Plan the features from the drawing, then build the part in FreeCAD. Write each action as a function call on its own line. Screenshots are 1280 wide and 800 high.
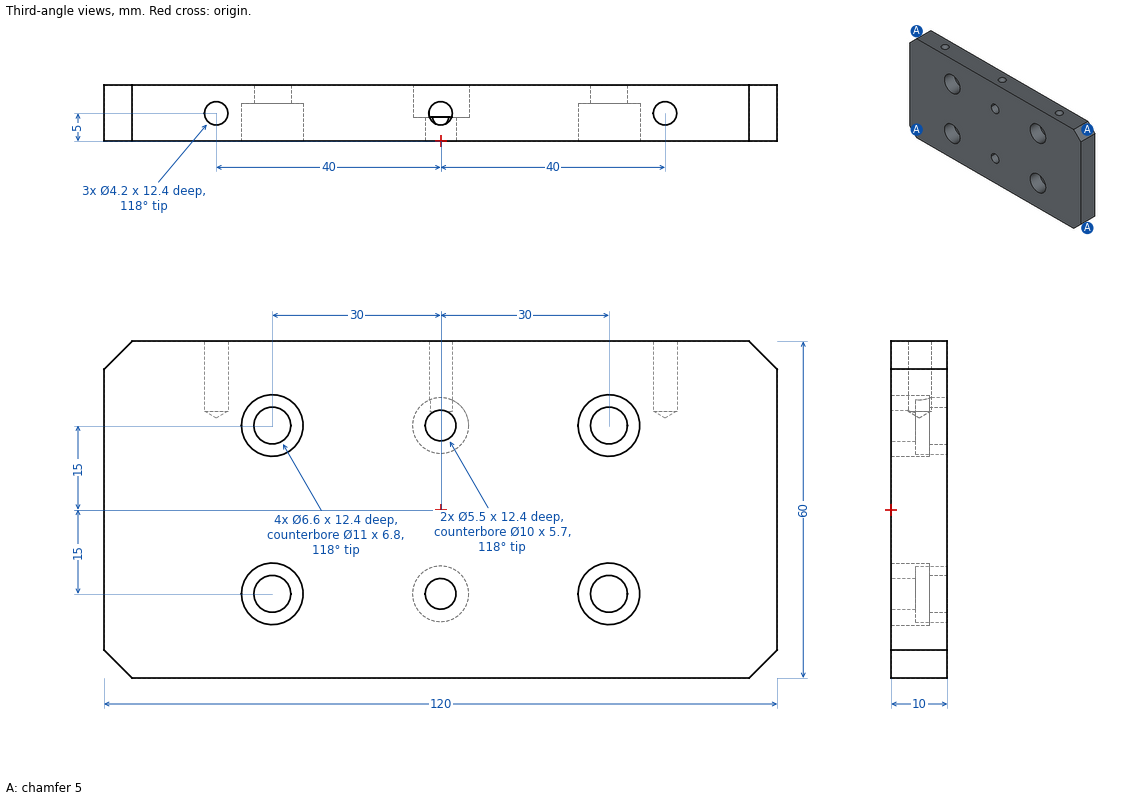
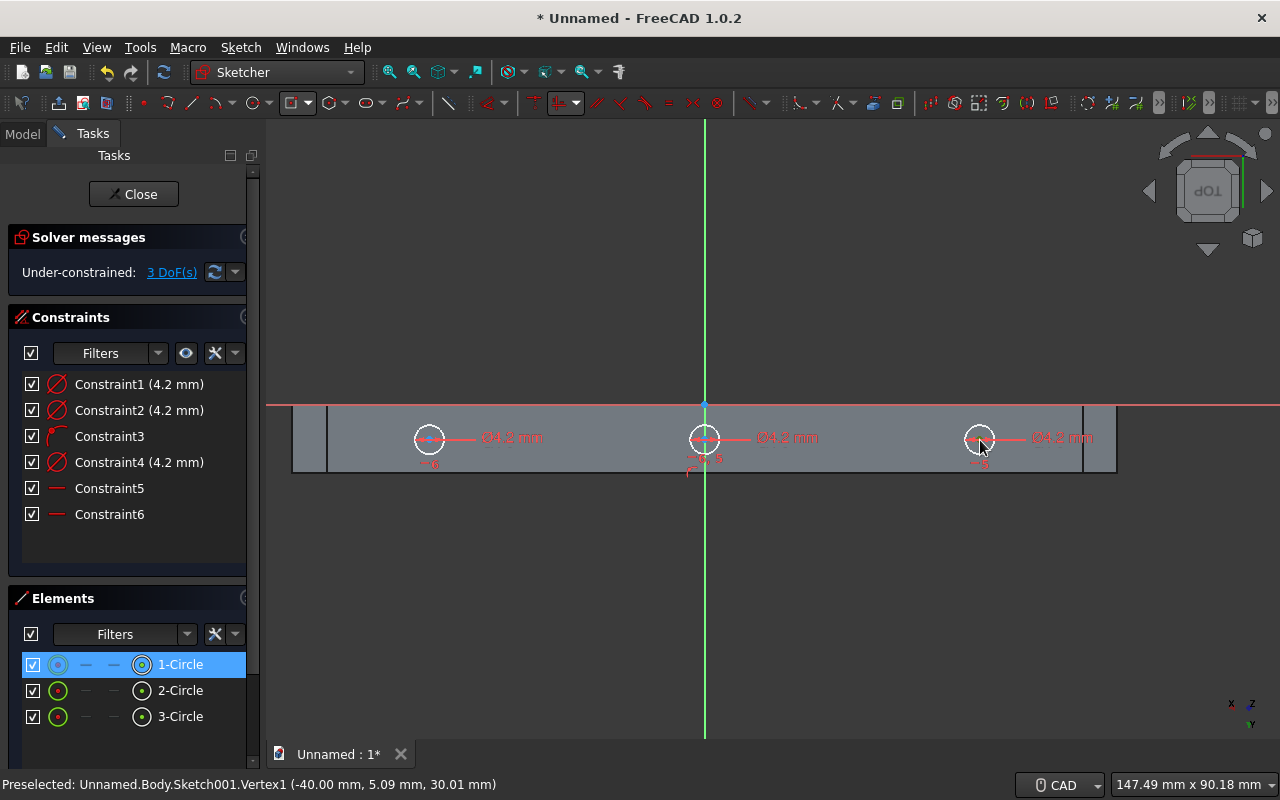
key(i)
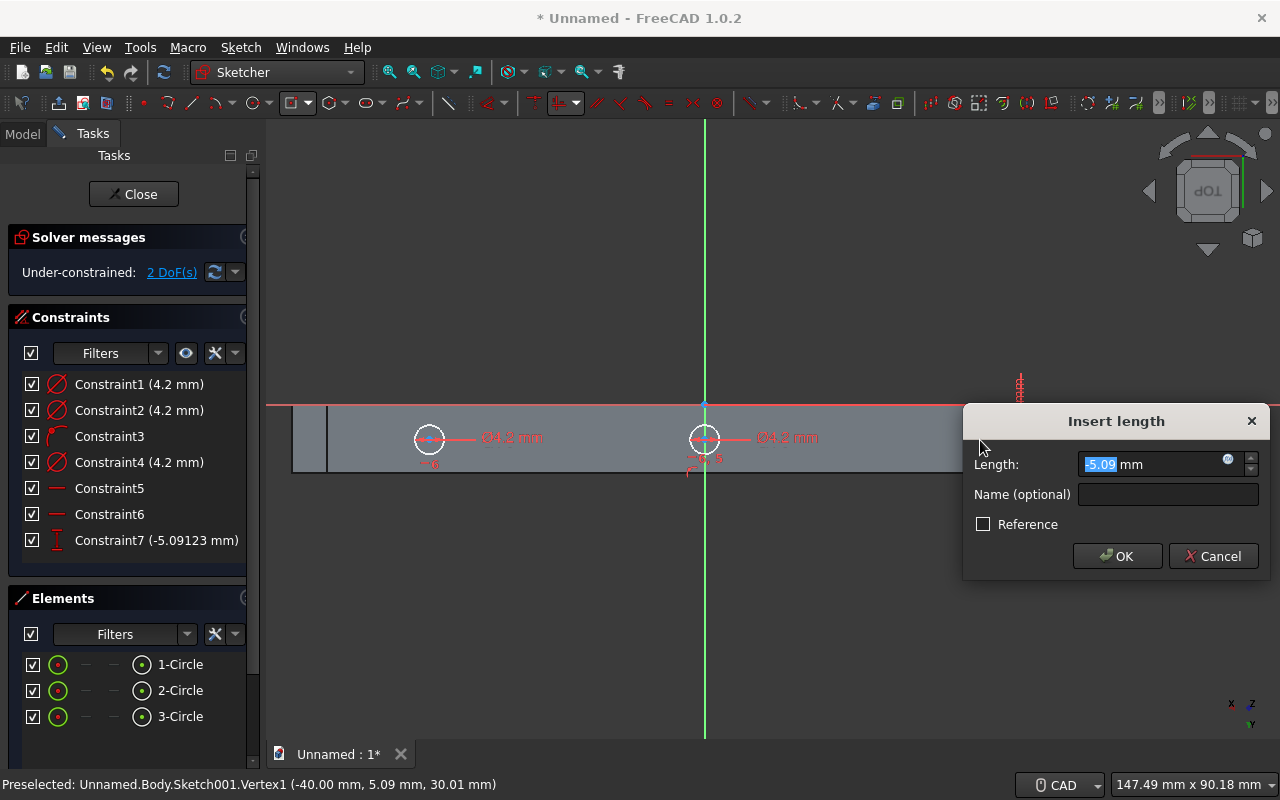
text(-5)
key(Return)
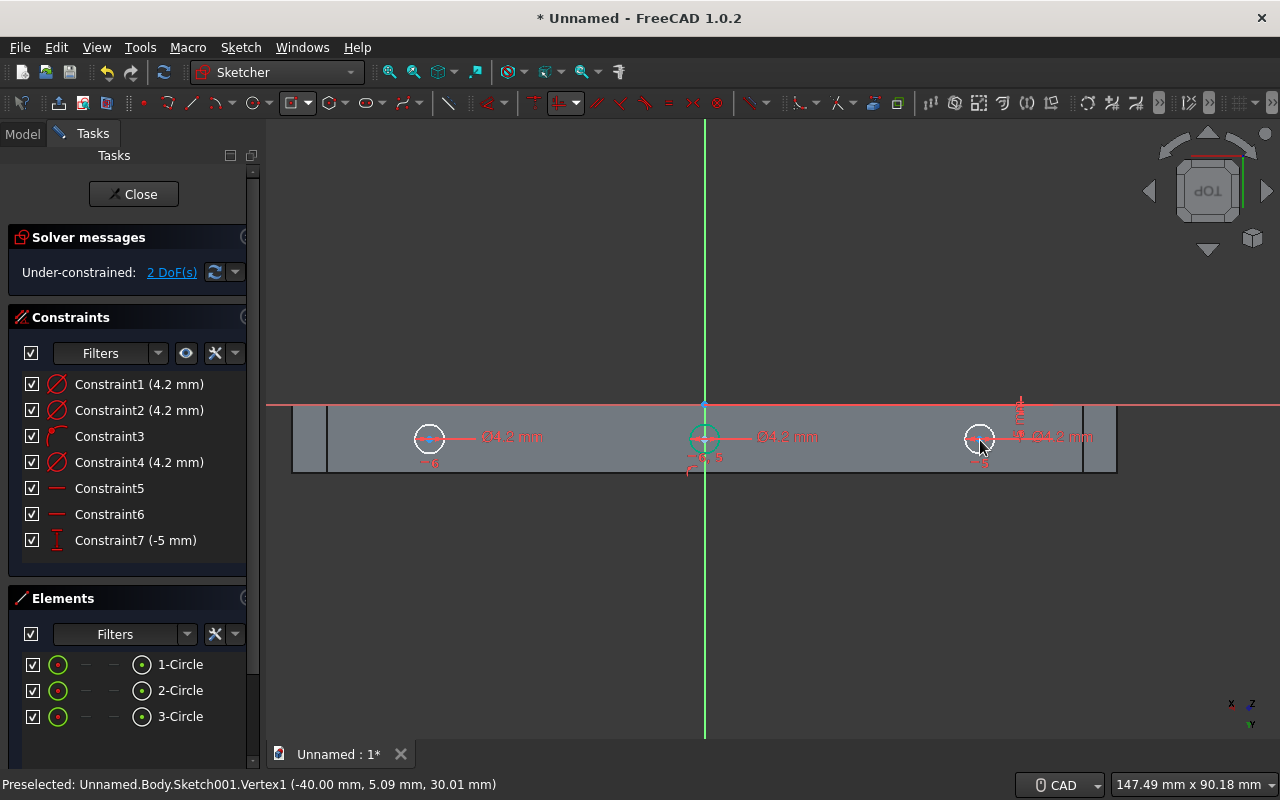
click(980, 439)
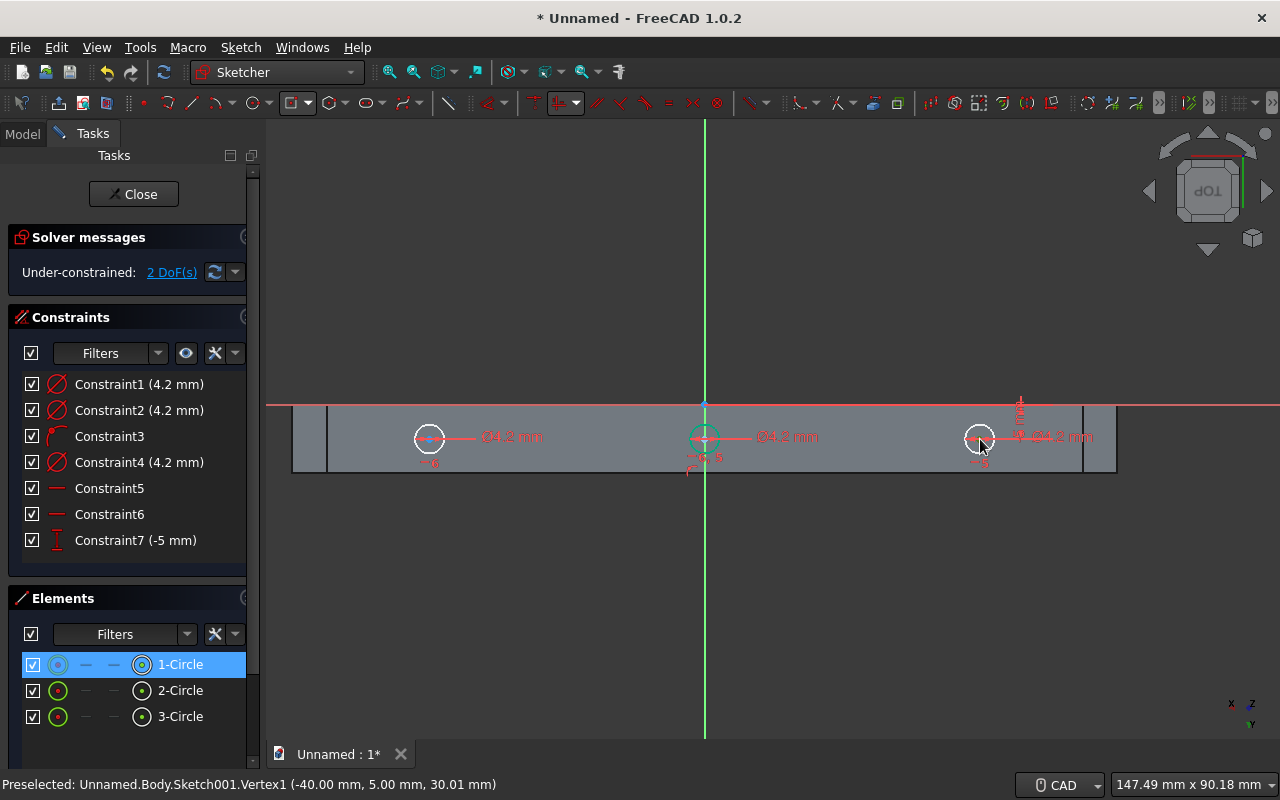
key(l)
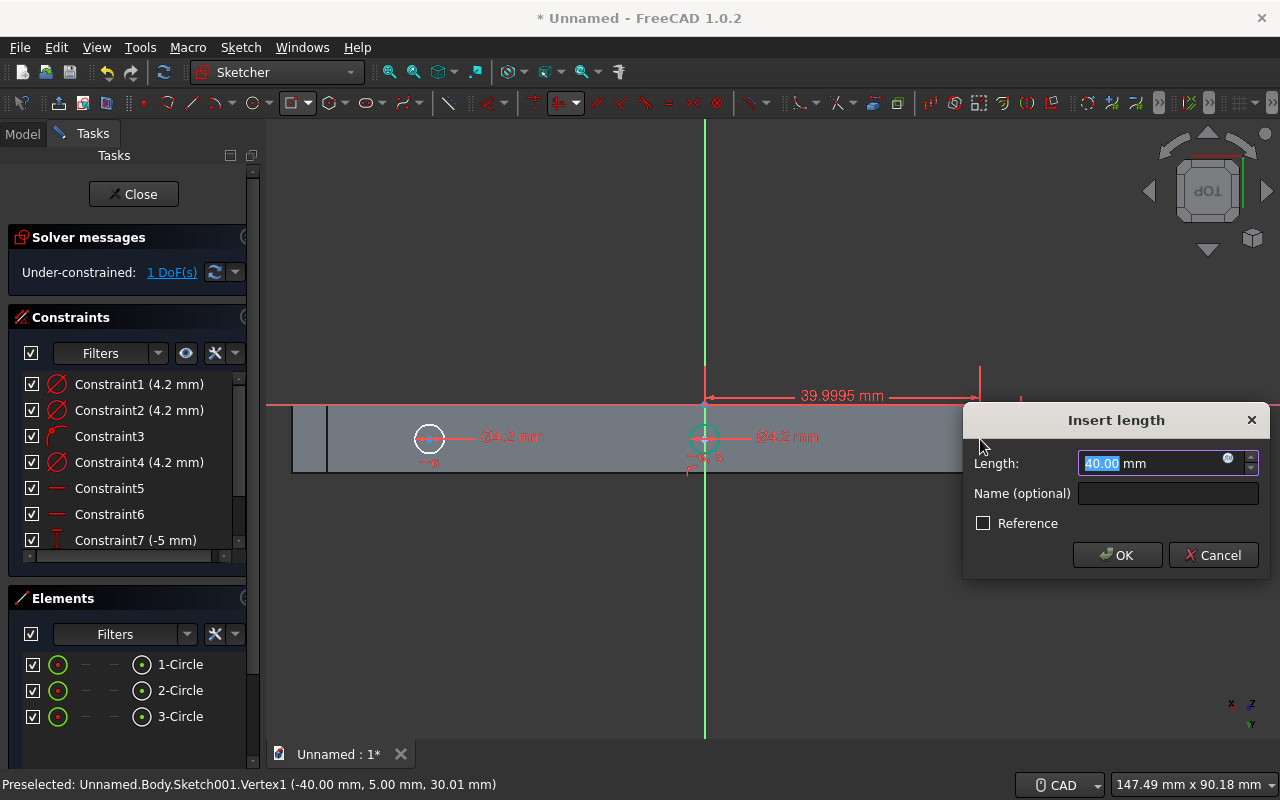
text(40)
key(Return)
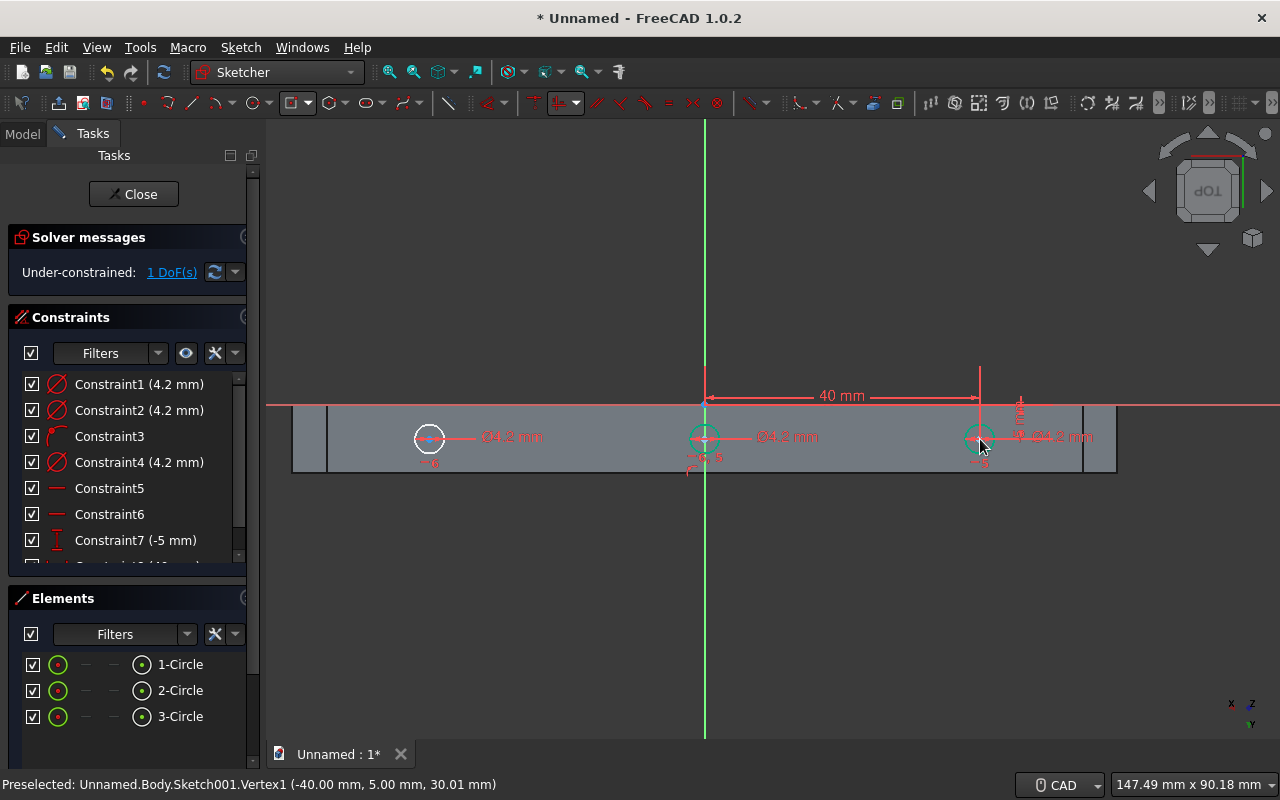
click(430, 439)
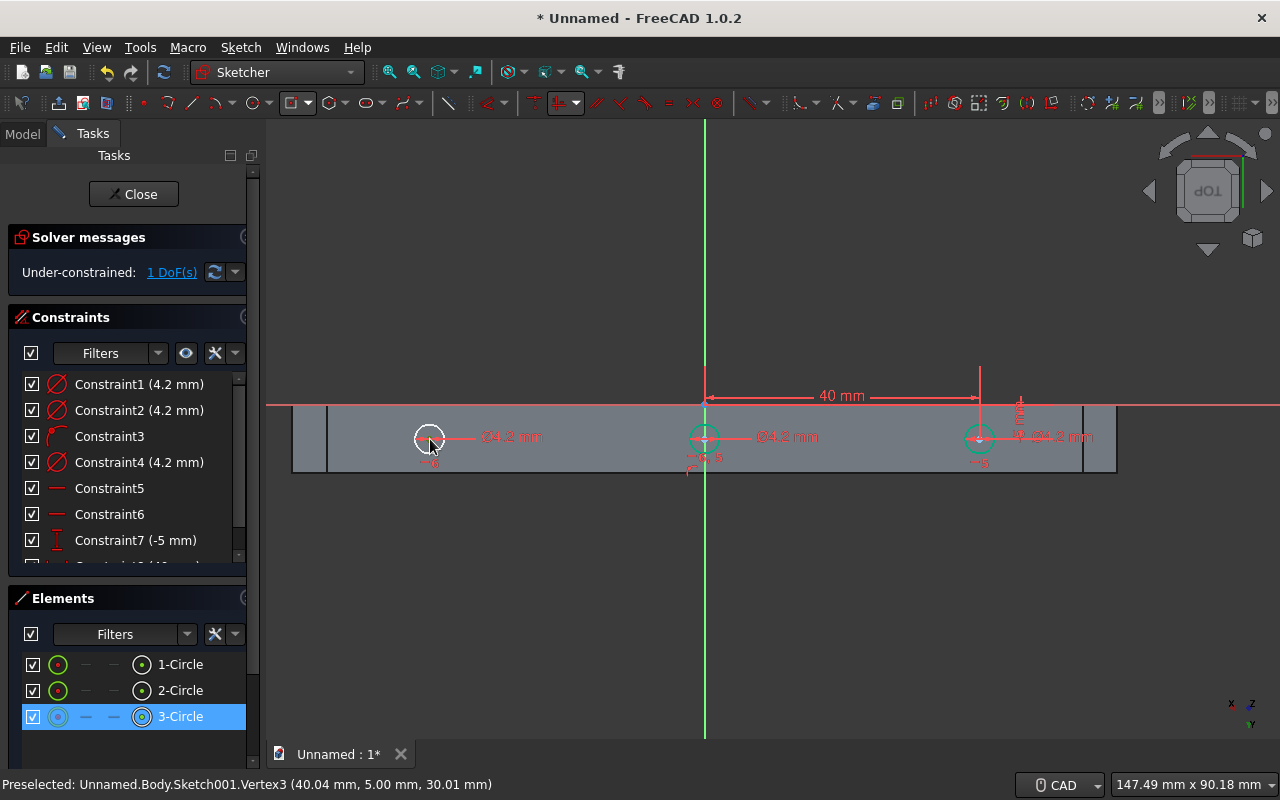
key(l)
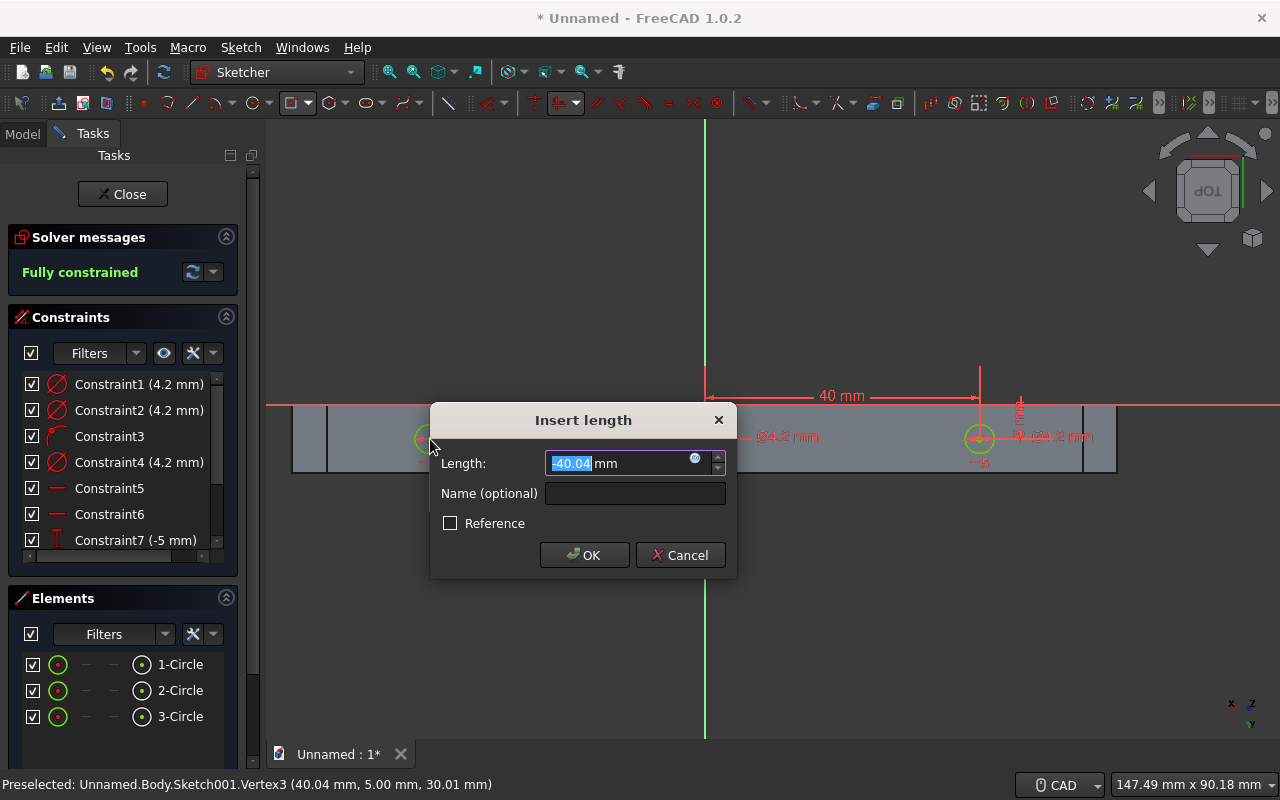
text(-40)
key(Return)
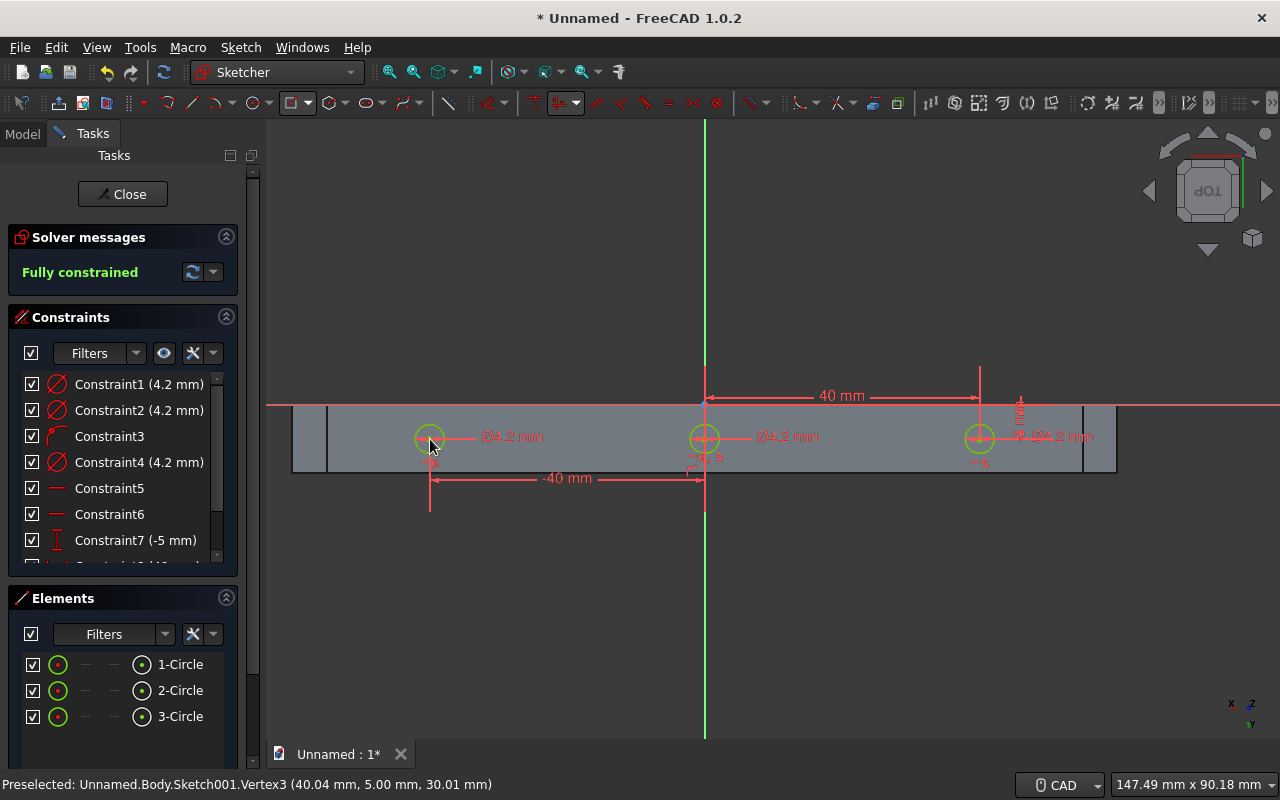
click(123, 194)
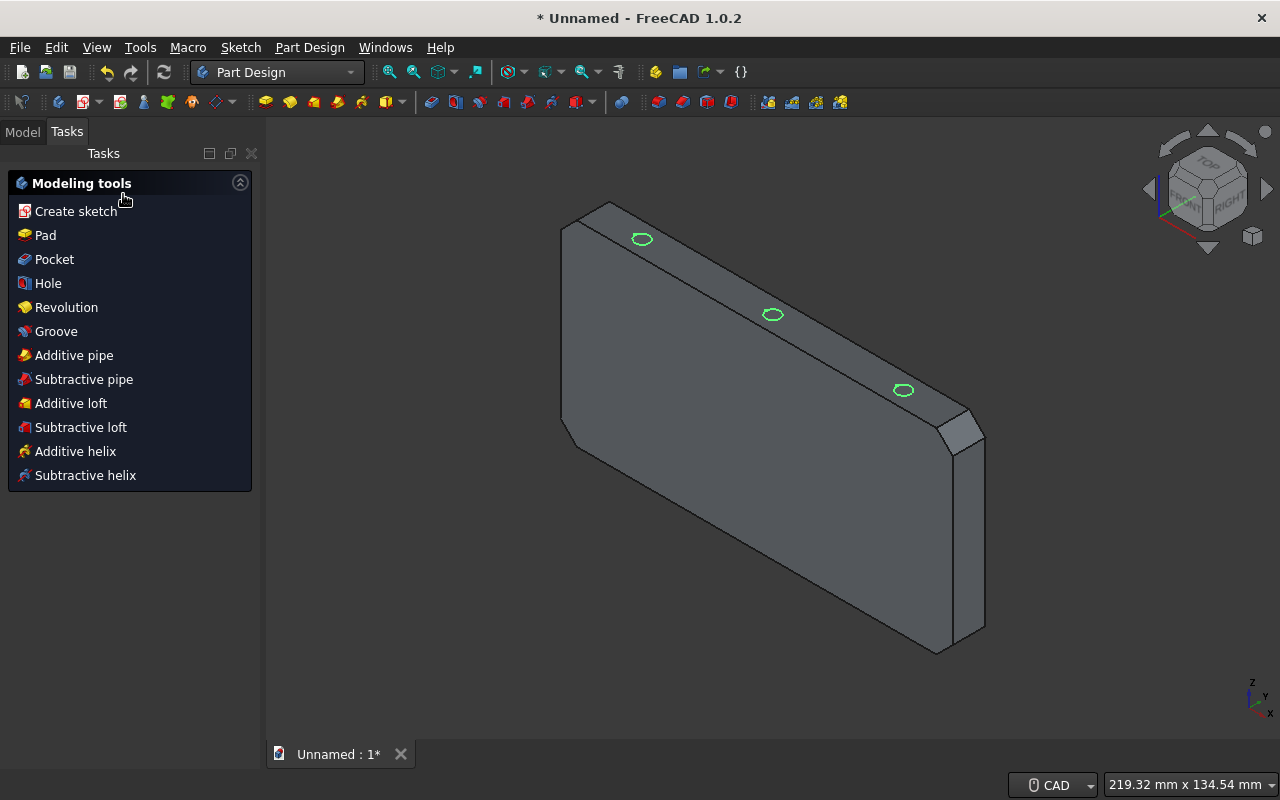
click(456, 102)